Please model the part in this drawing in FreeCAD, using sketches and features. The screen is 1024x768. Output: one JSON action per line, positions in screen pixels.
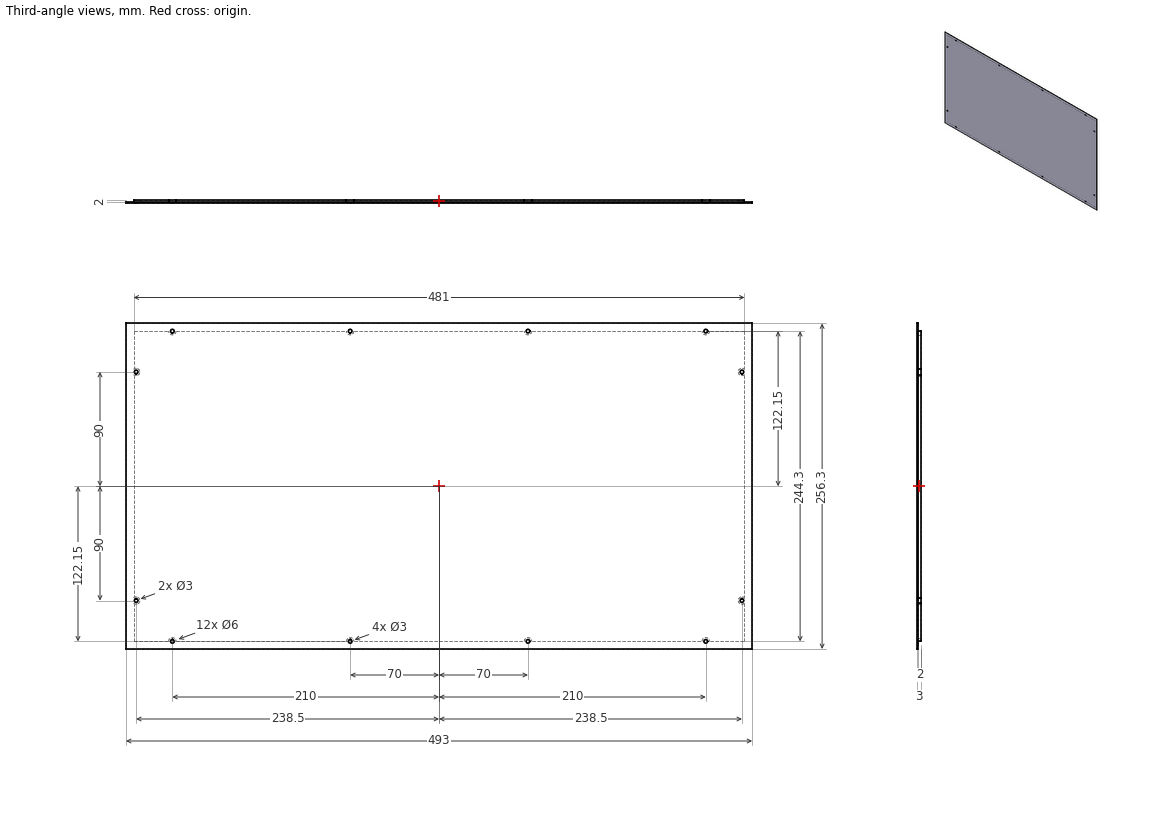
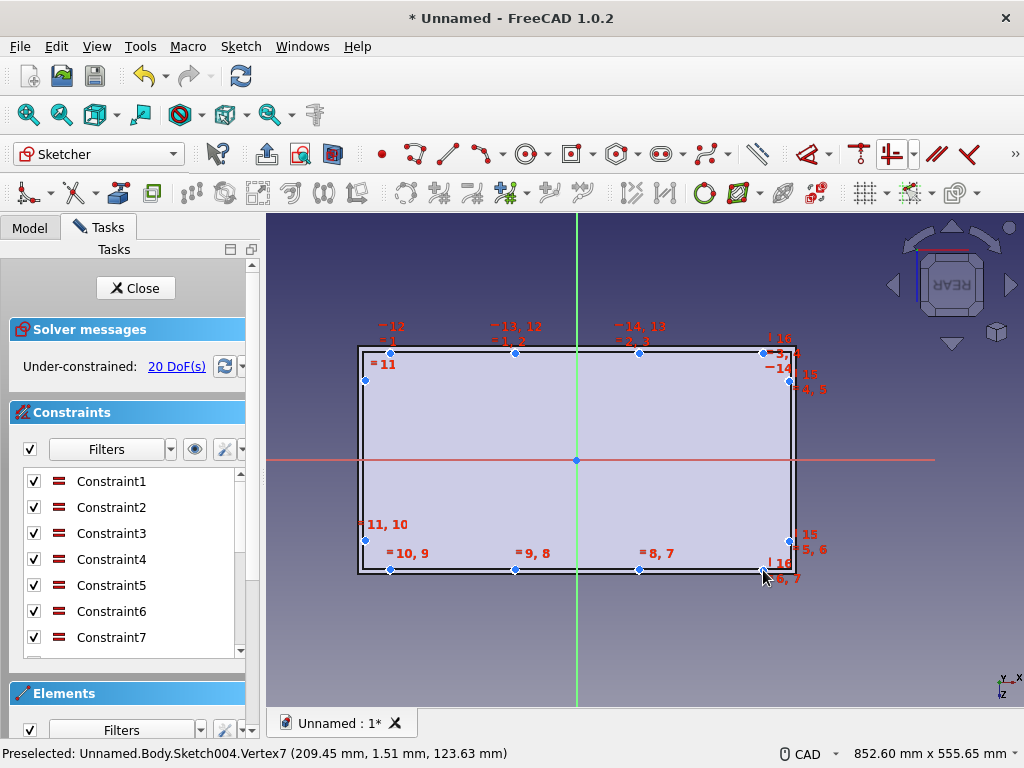
{"action": "left_click", "coordinate": [639, 353]}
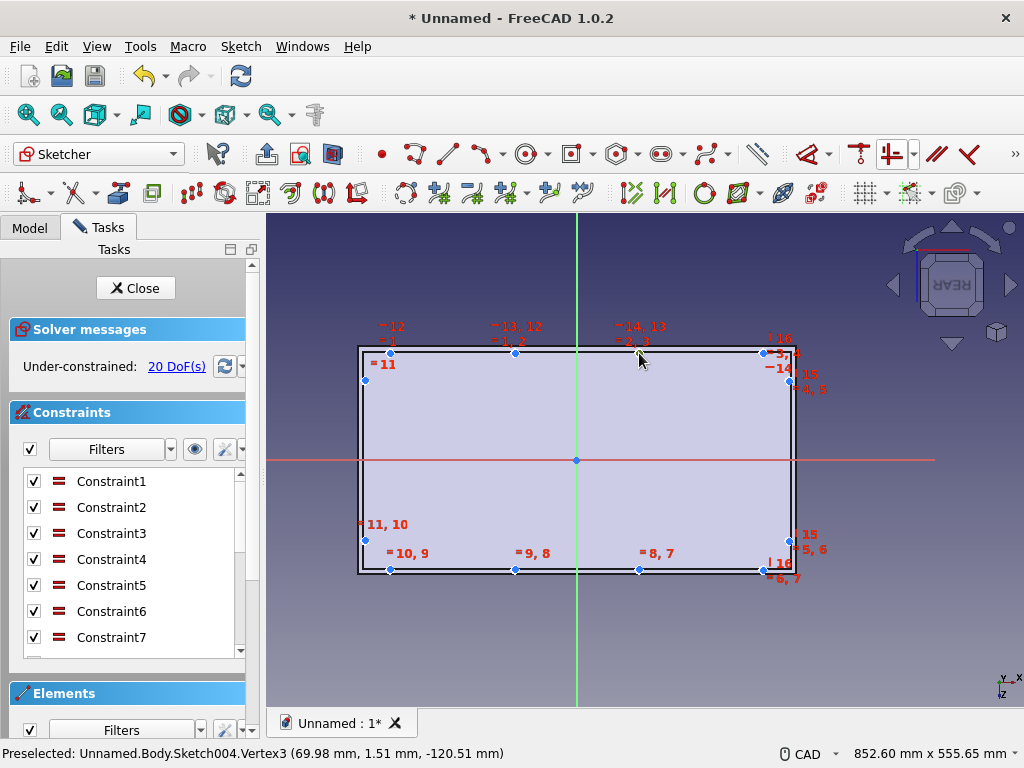
{"action": "left_click", "coordinate": [639, 570]}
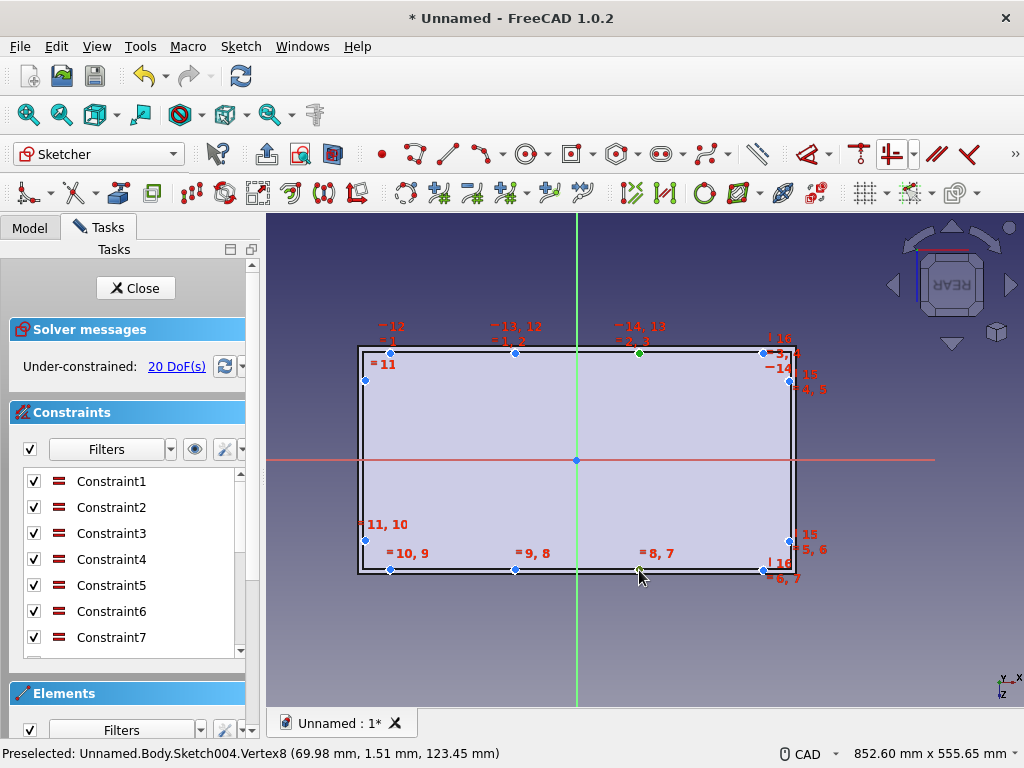
{"action": "key", "text": "v"}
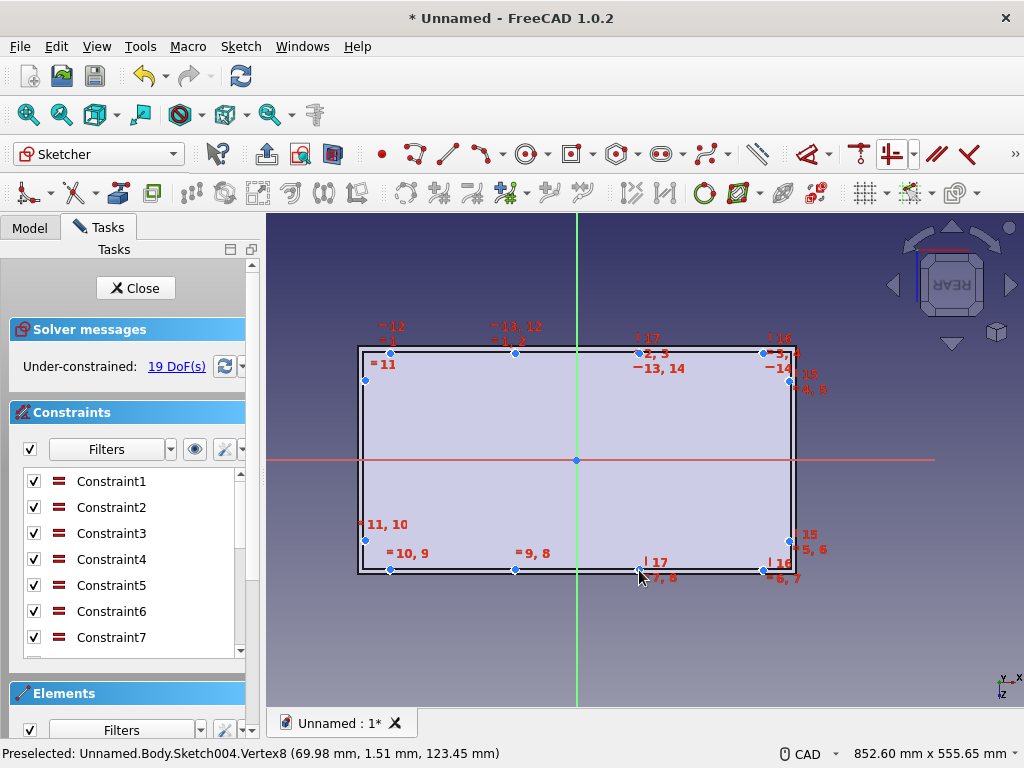
{"action": "left_click", "coordinate": [763, 570]}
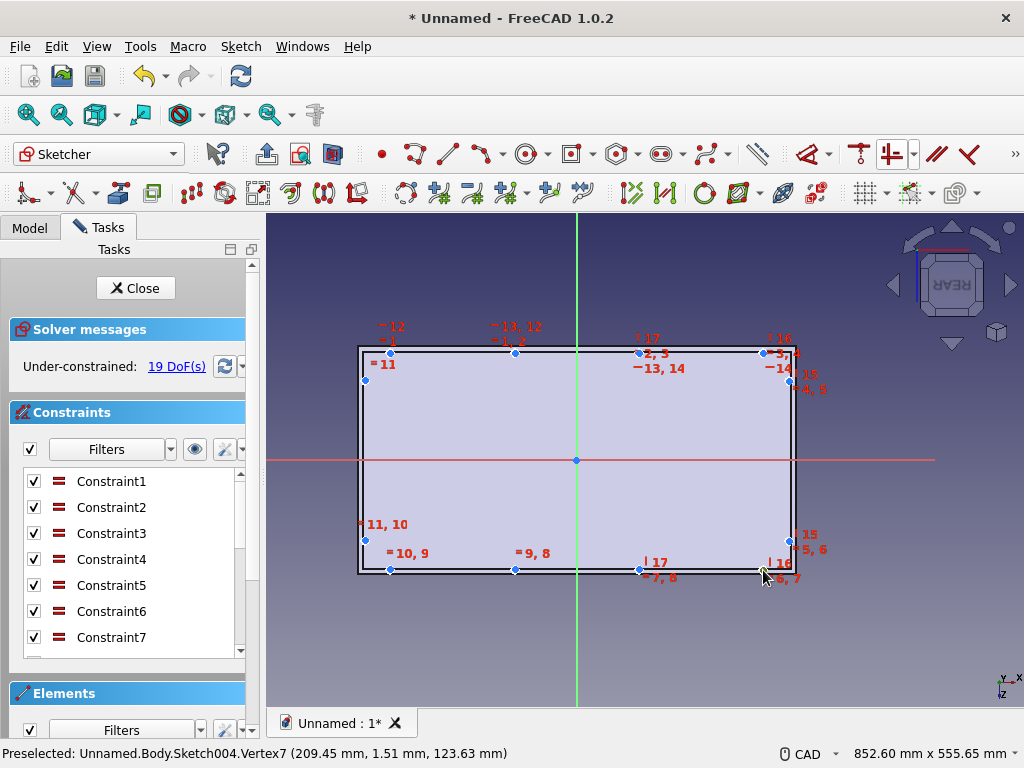
{"action": "left_click", "coordinate": [639, 570]}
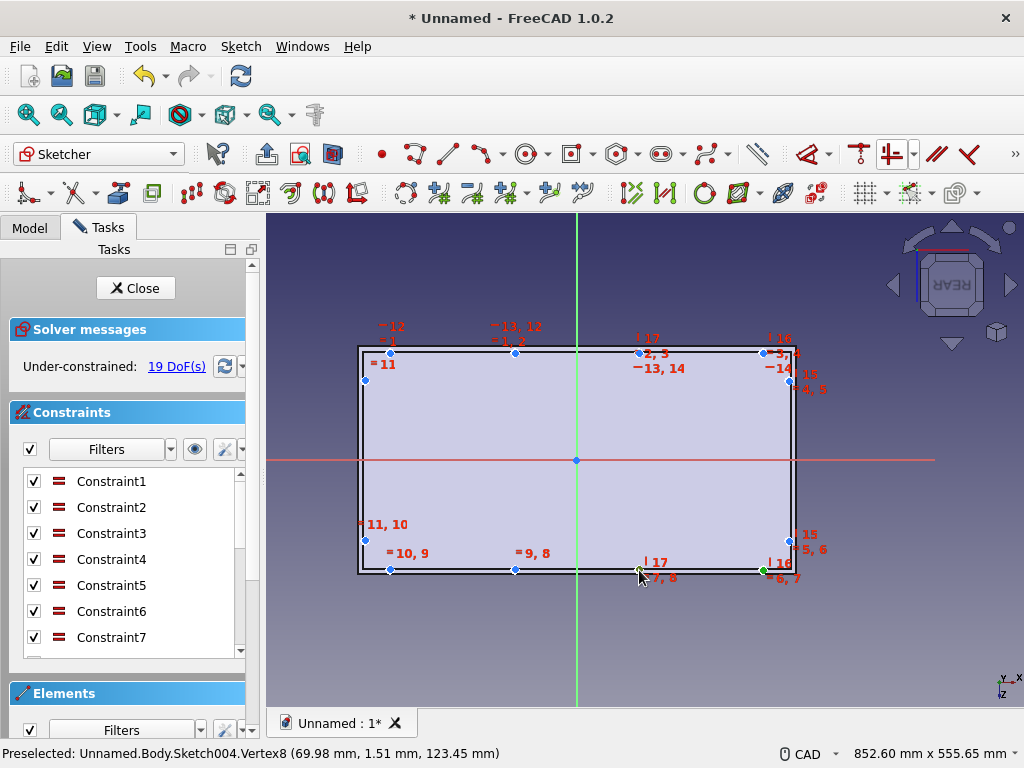
{"action": "key", "text": "h"}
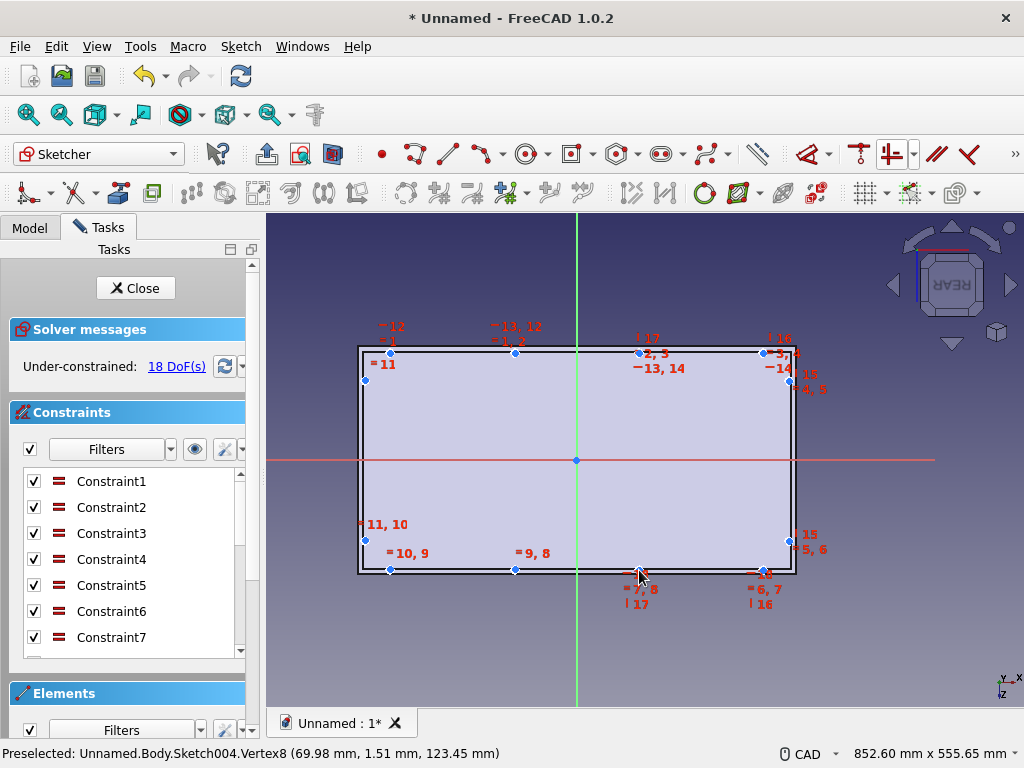
{"action": "left_click", "coordinate": [515, 353]}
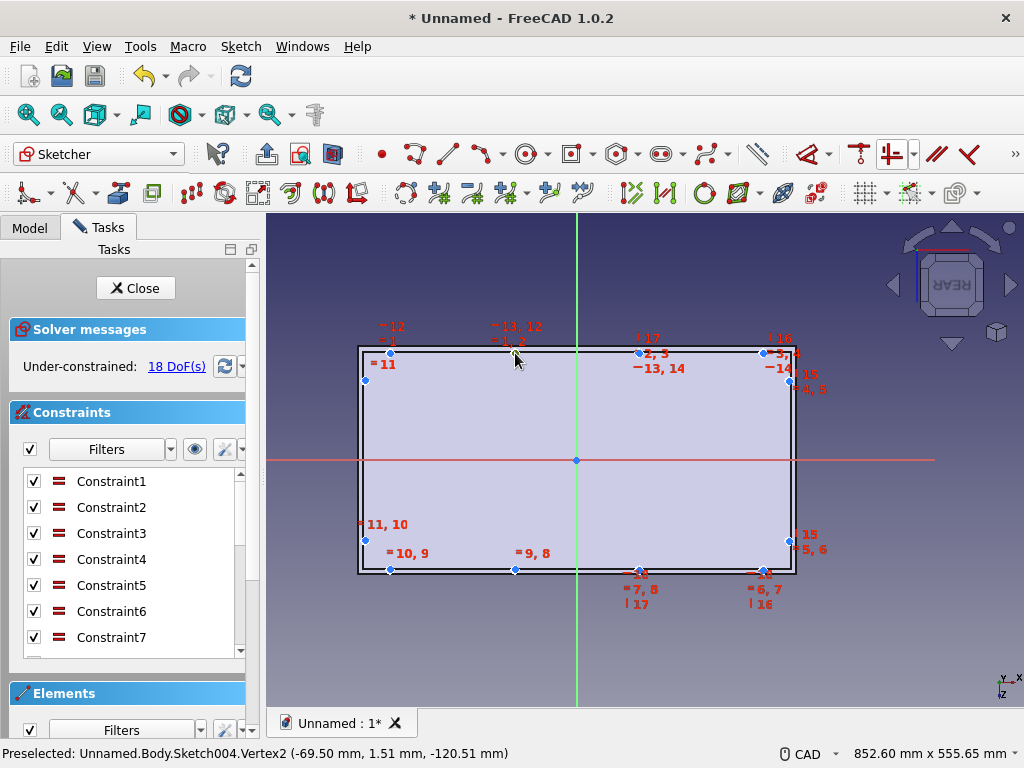
{"action": "left_click", "coordinate": [515, 570]}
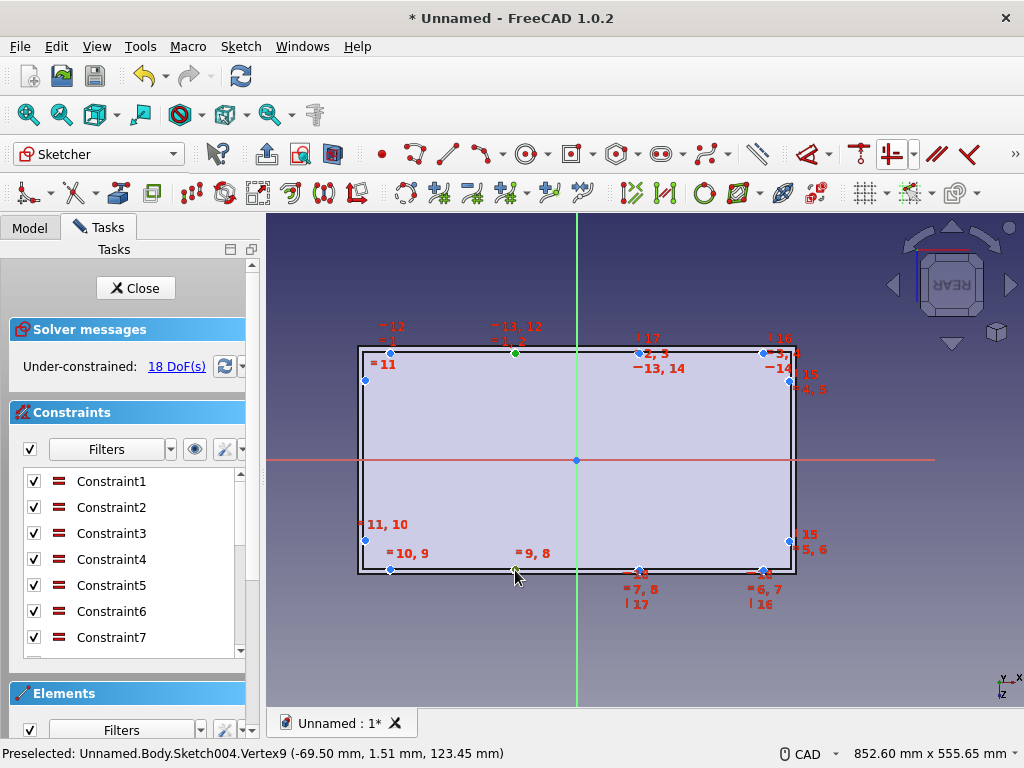
{"action": "key", "text": "v"}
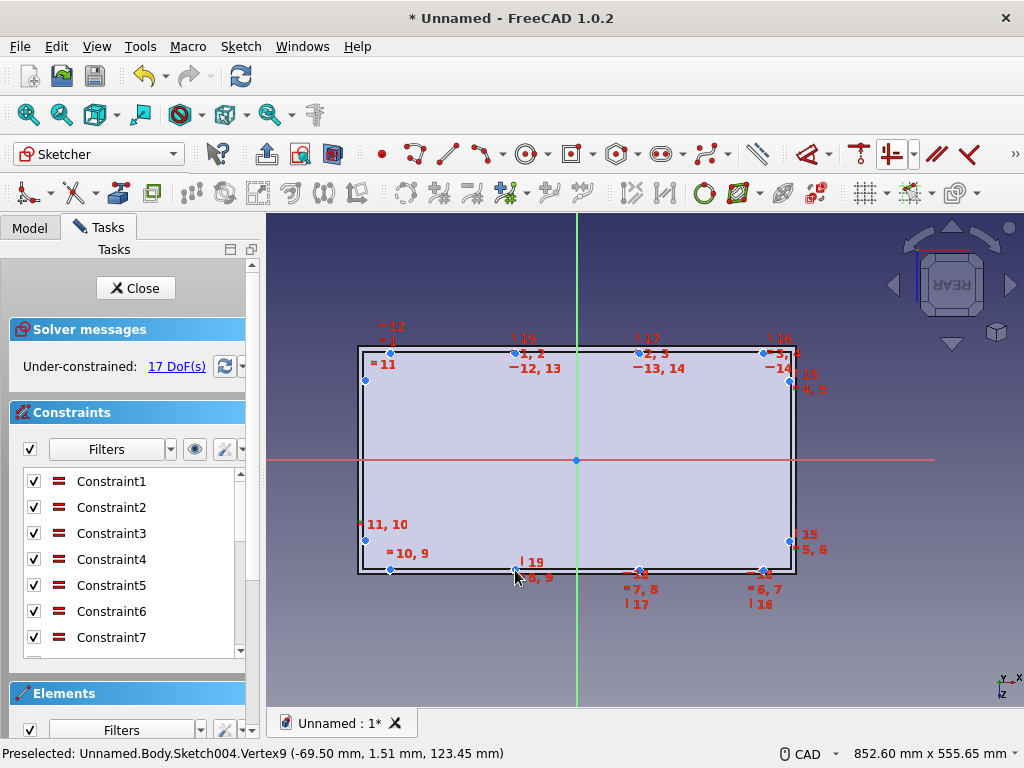
{"action": "scroll", "coordinate": [639, 570], "scroll_direction": "up", "scroll_amount": 4}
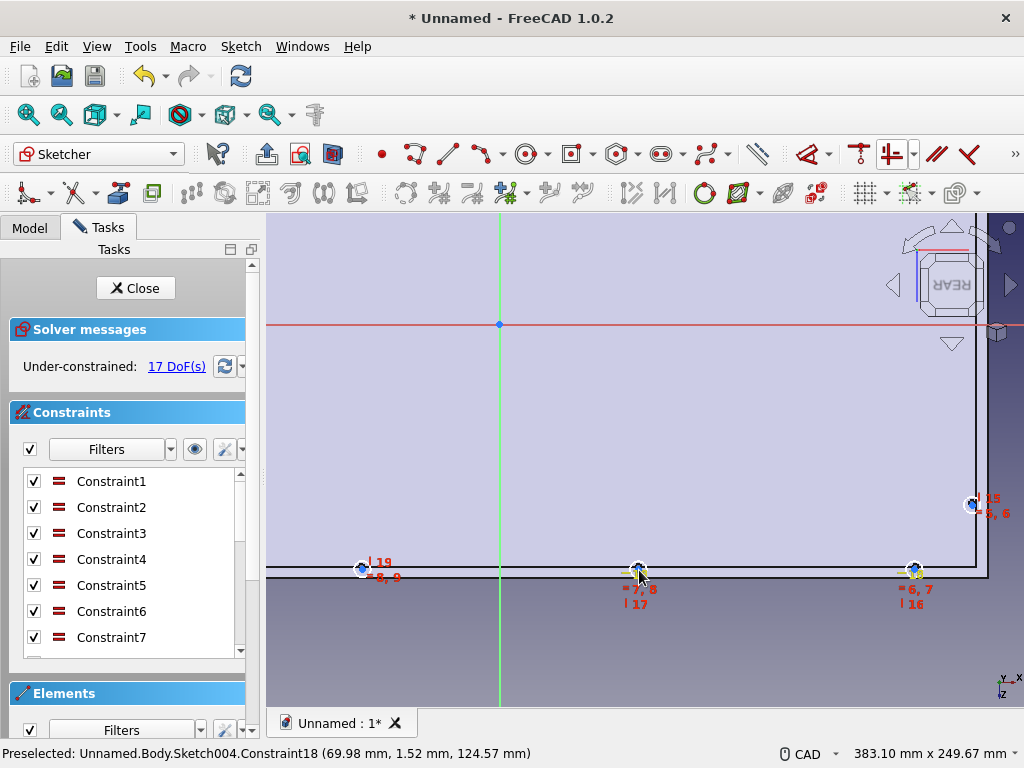
{"action": "scroll", "coordinate": [638, 569], "scroll_direction": "up", "scroll_amount": 4}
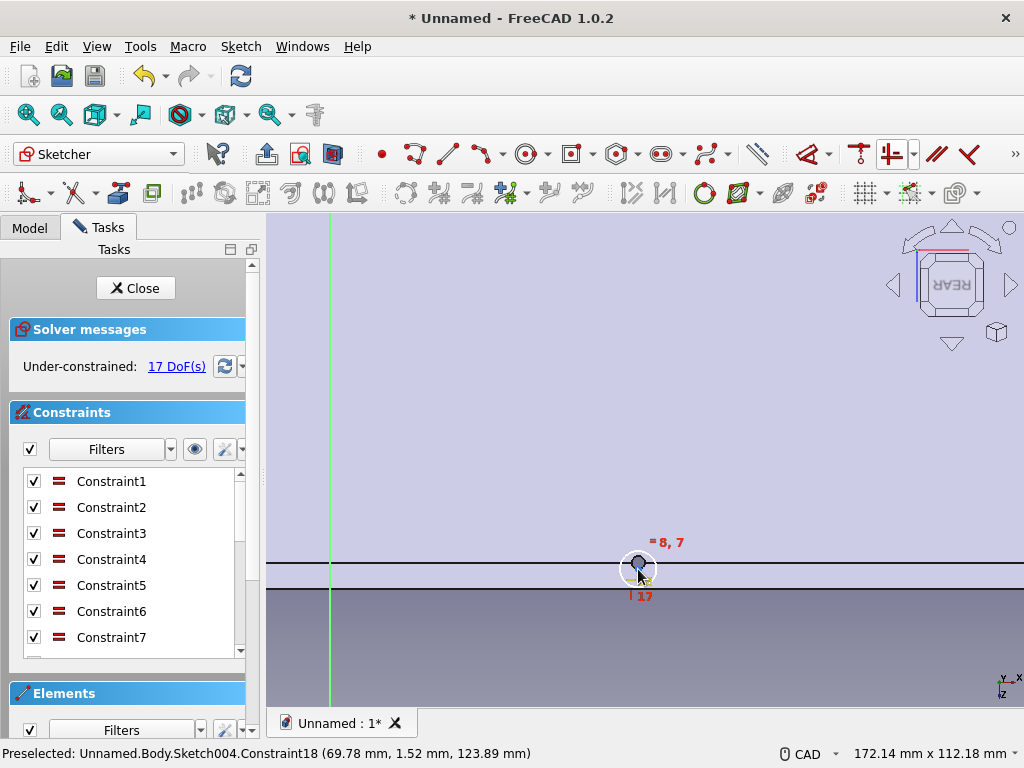
{"action": "left_click", "coordinate": [638, 569]}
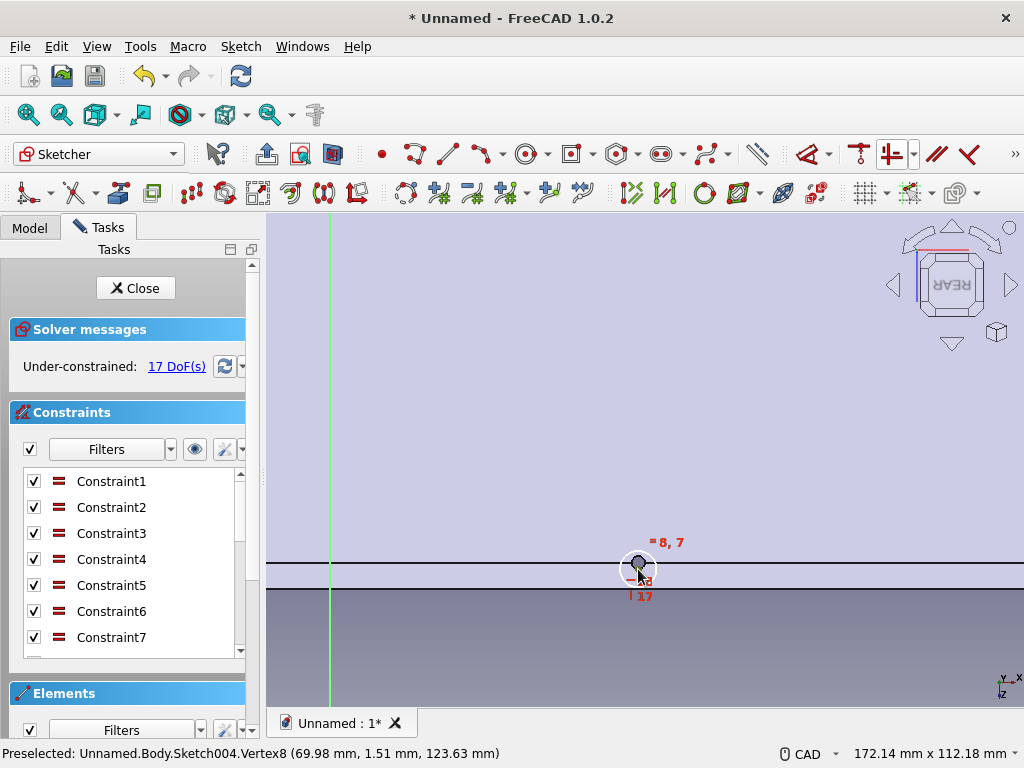
{"action": "scroll", "coordinate": [639, 570], "scroll_direction": "down", "scroll_amount": 8}